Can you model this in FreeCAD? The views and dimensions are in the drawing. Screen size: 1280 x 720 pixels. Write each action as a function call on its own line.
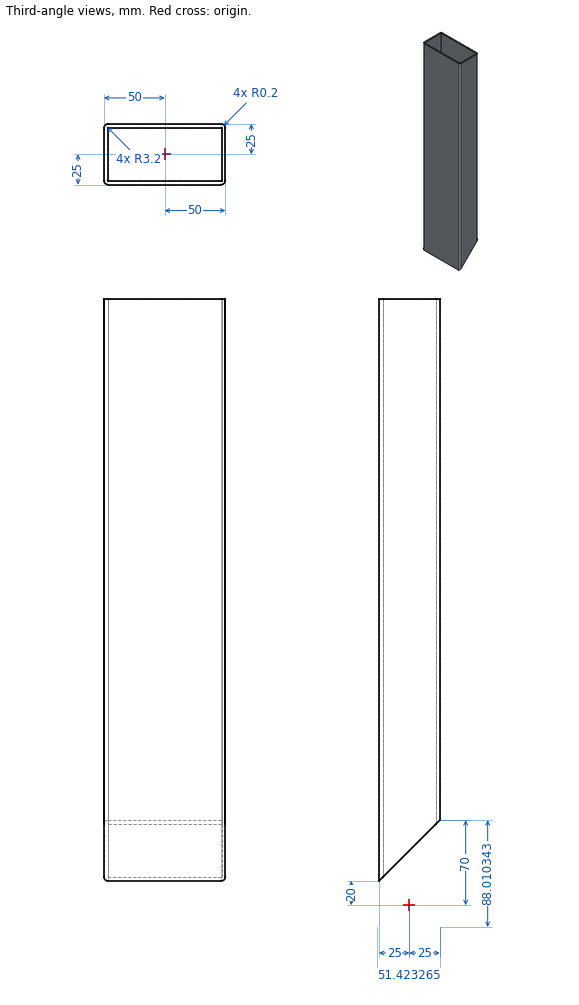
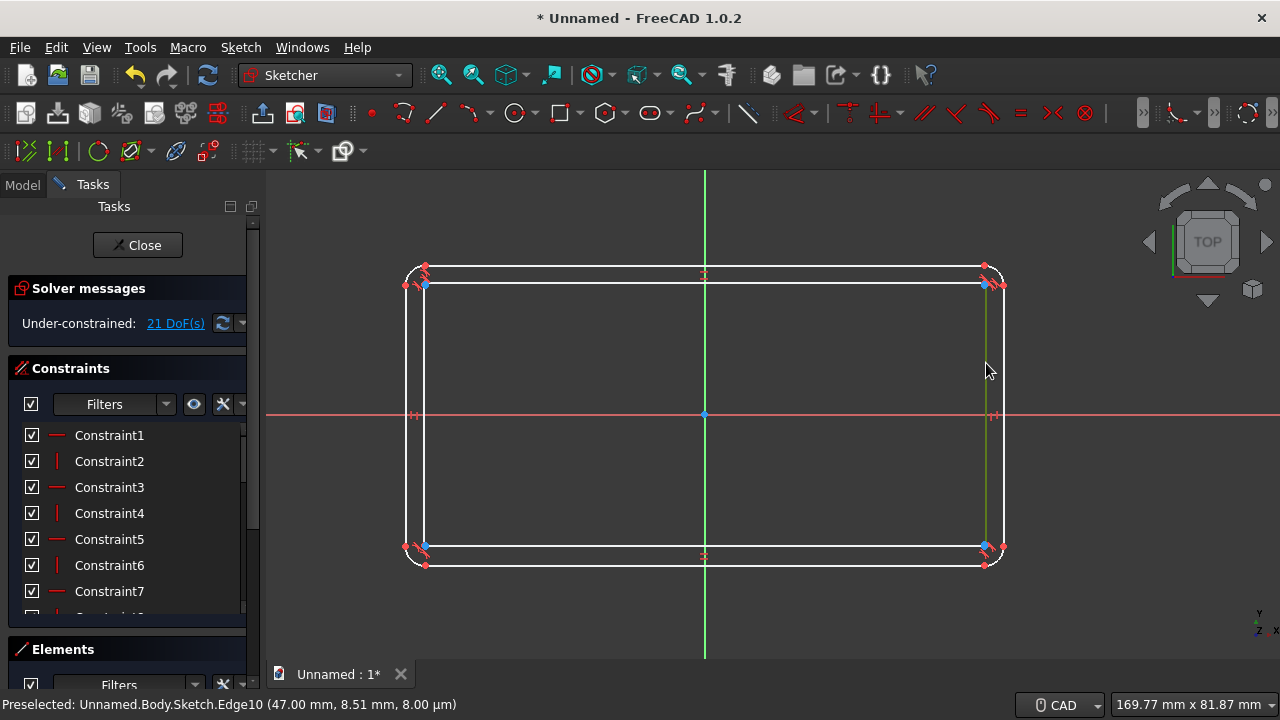
scroll(985, 546, up, 13)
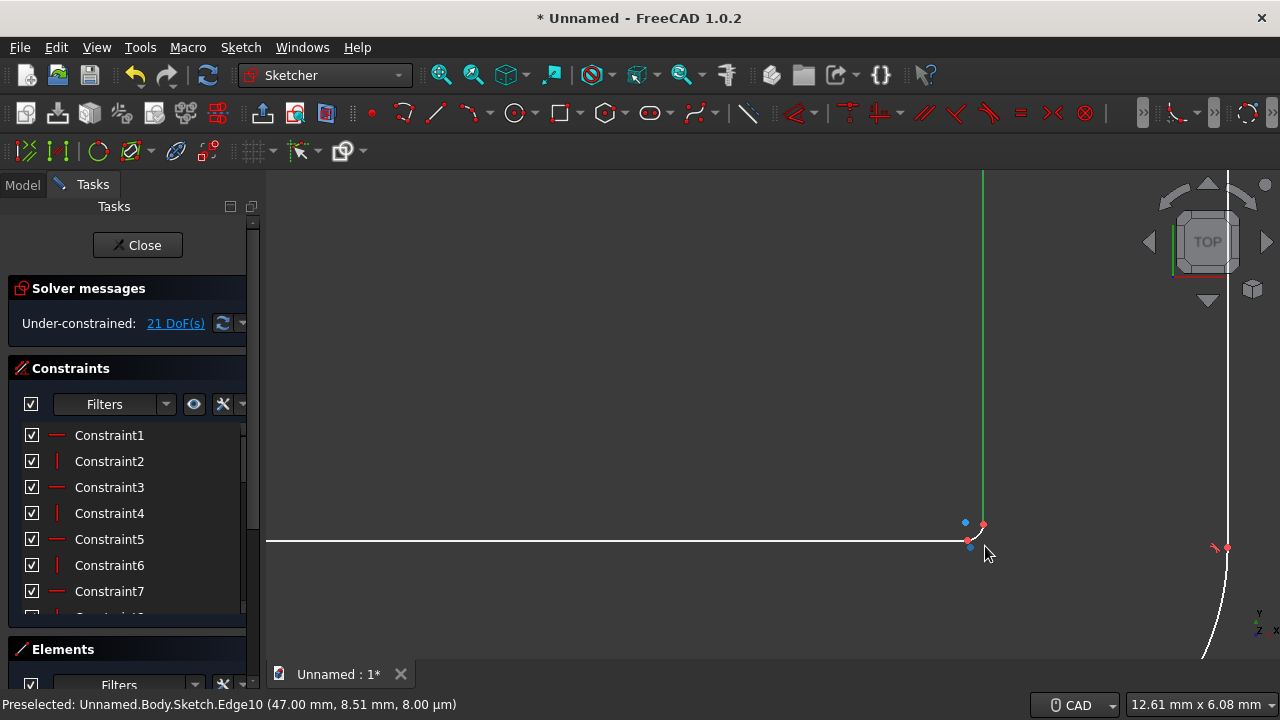
click(978, 536)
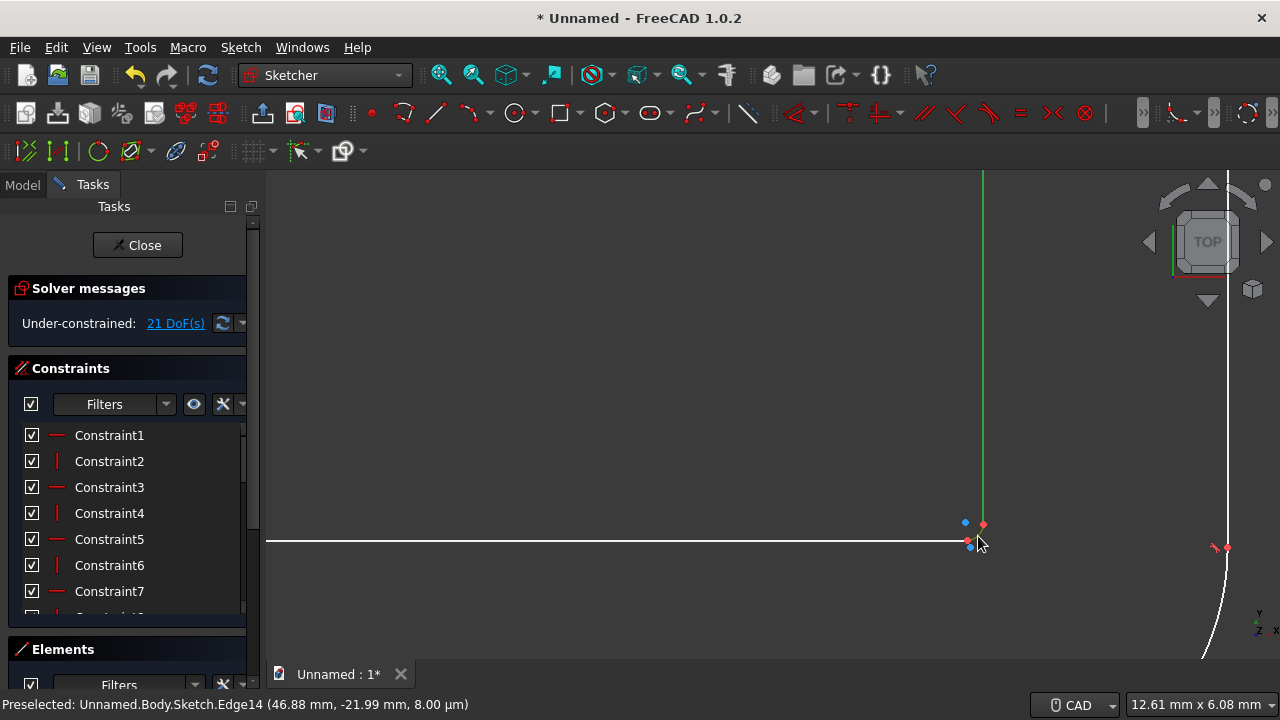
click(990, 114)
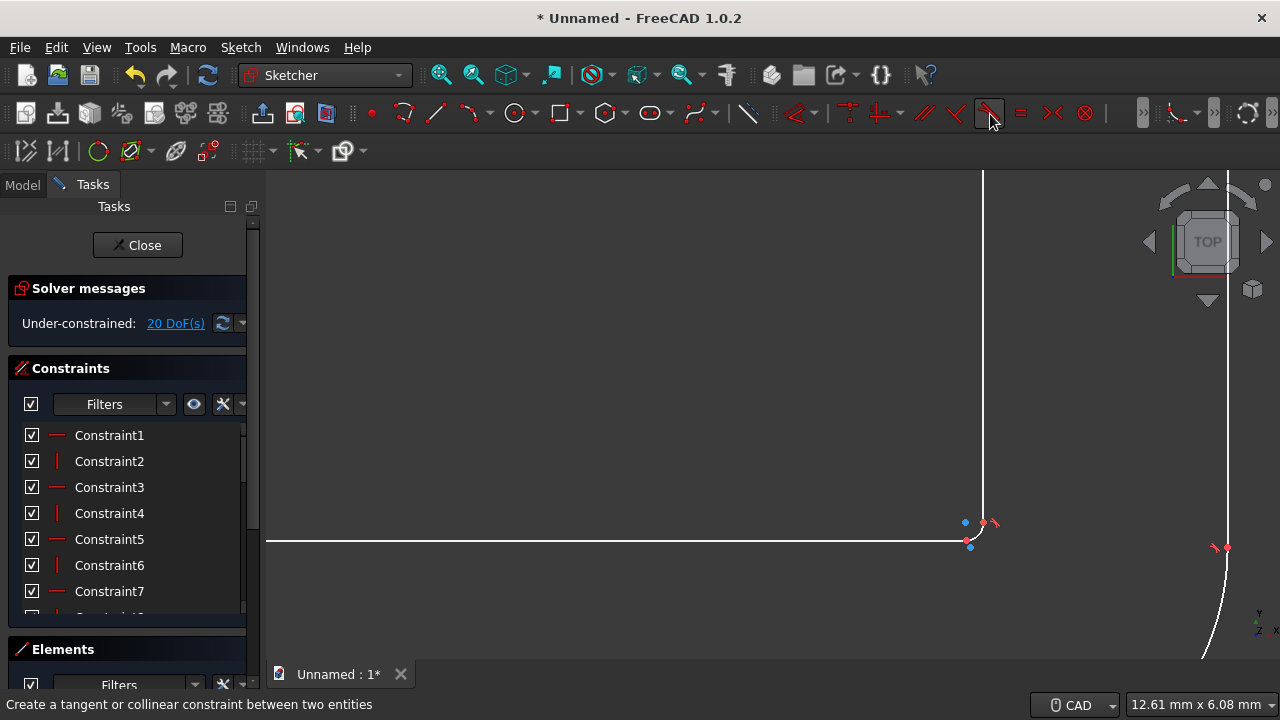
scroll(985, 546, down, 13)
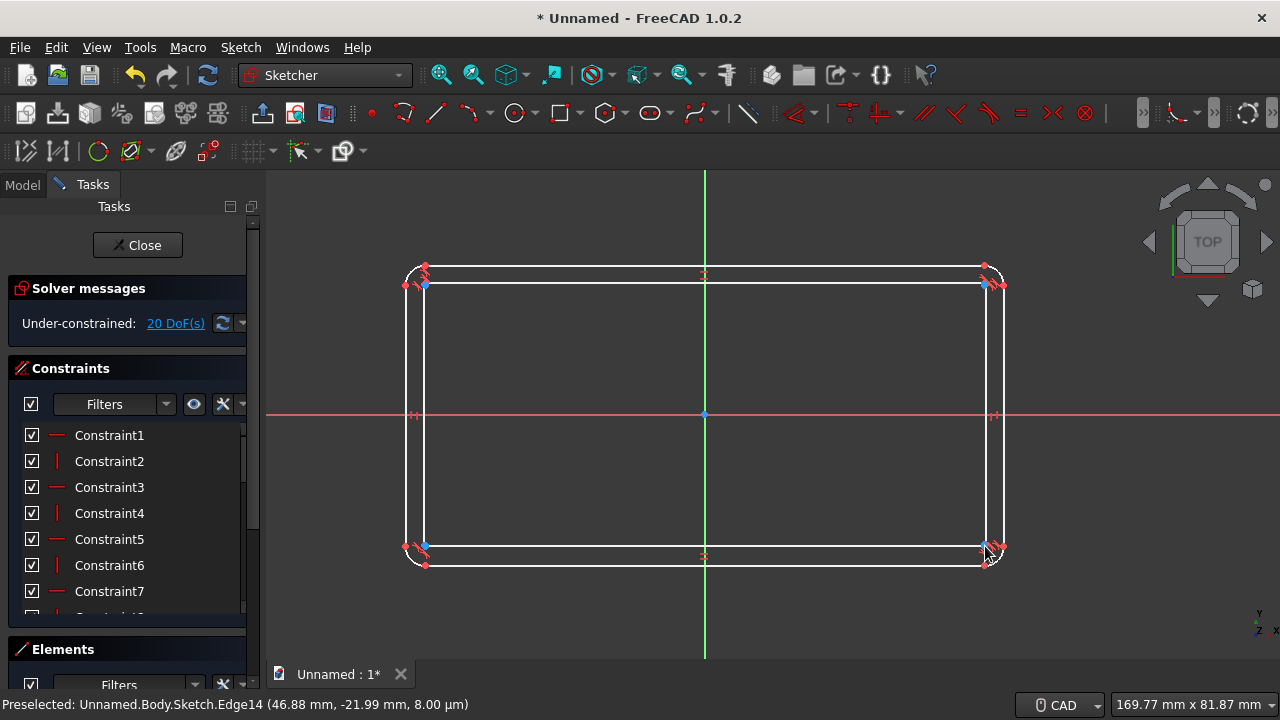
click(817, 546)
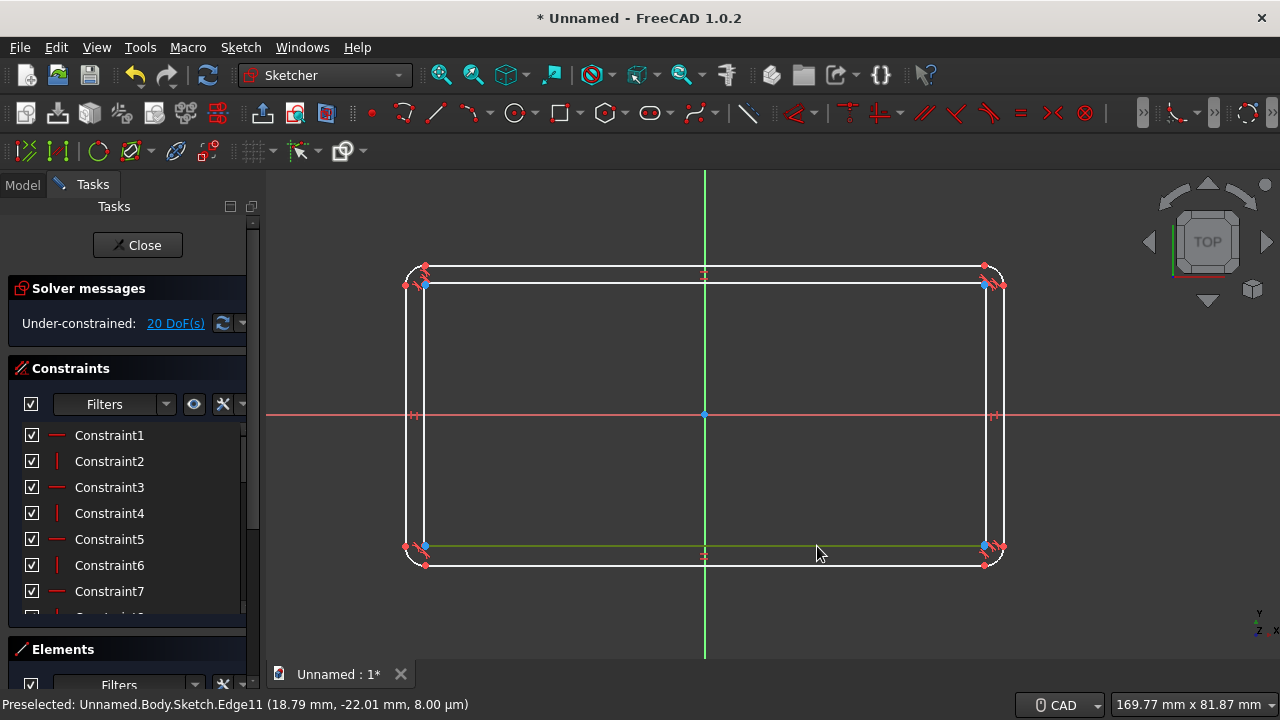
scroll(985, 546, up, 13)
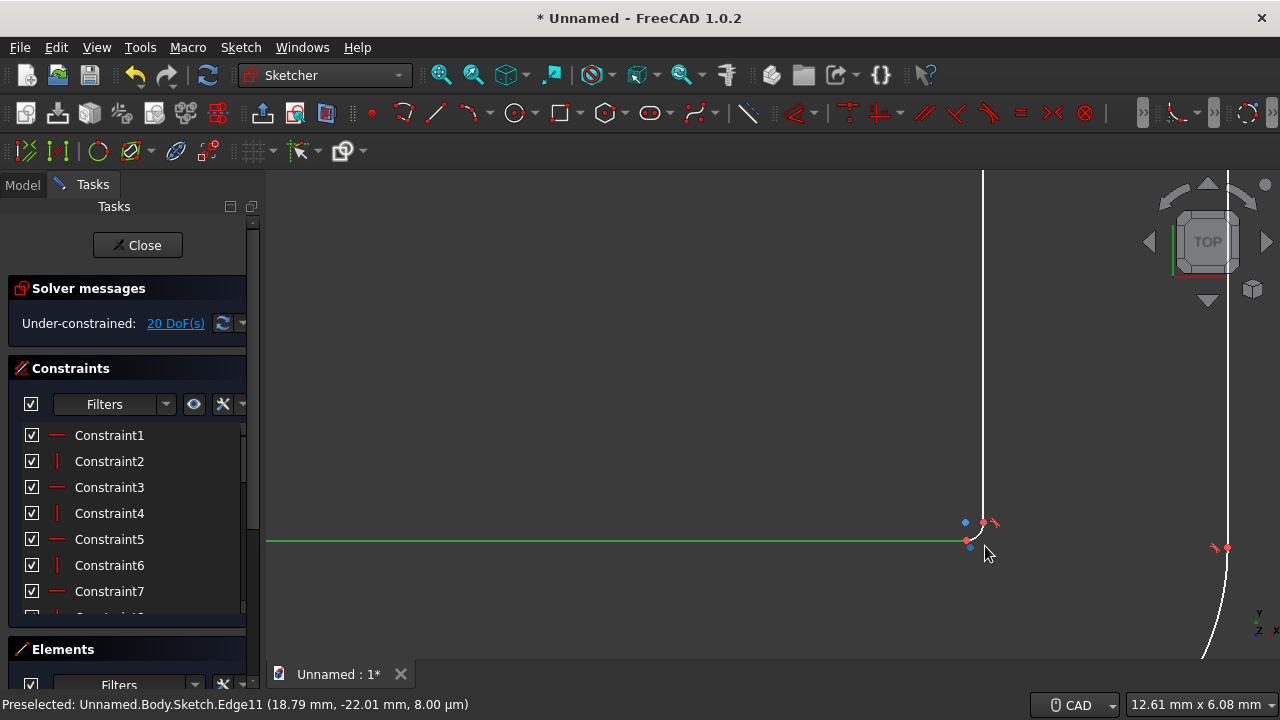
click(979, 535)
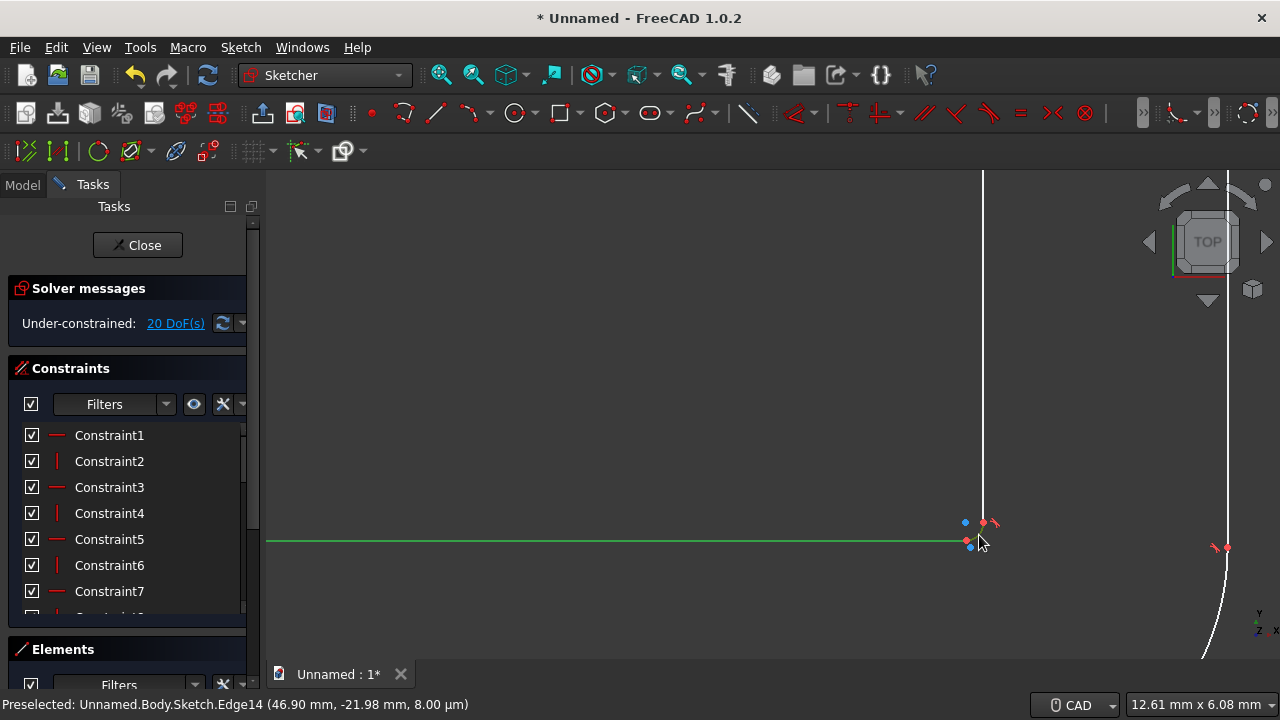
click(990, 114)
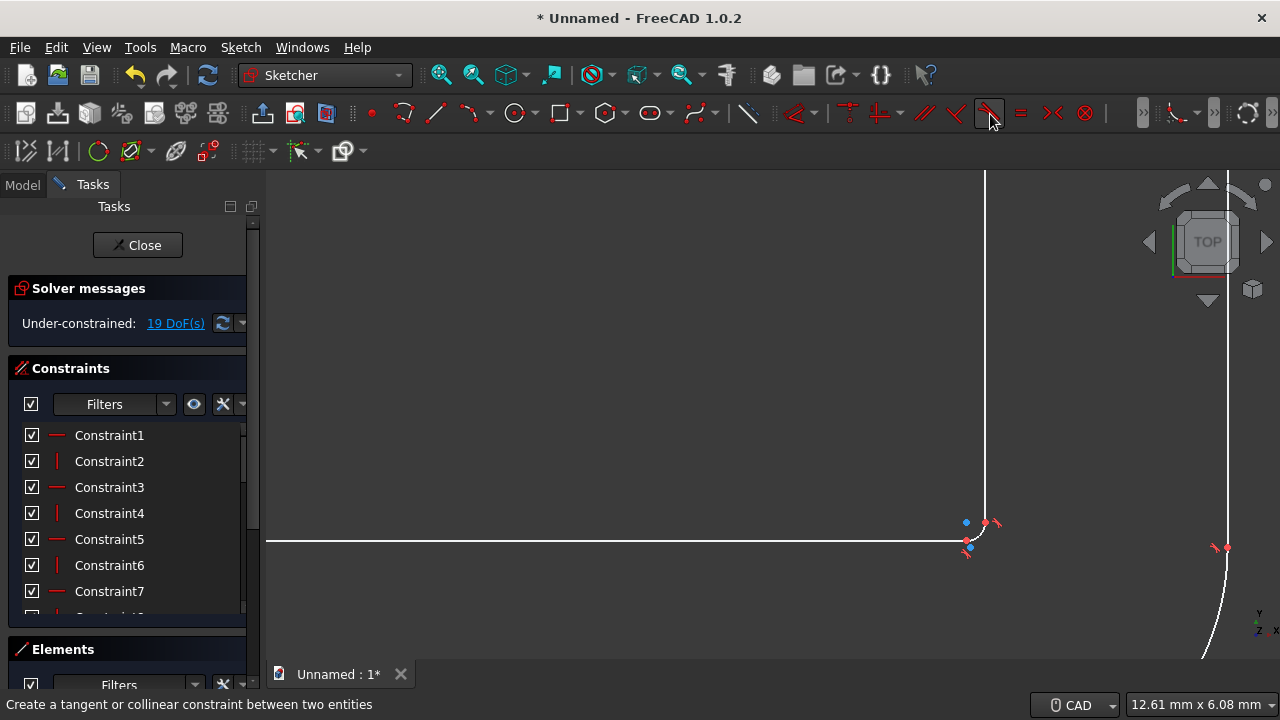
scroll(985, 546, down, 13)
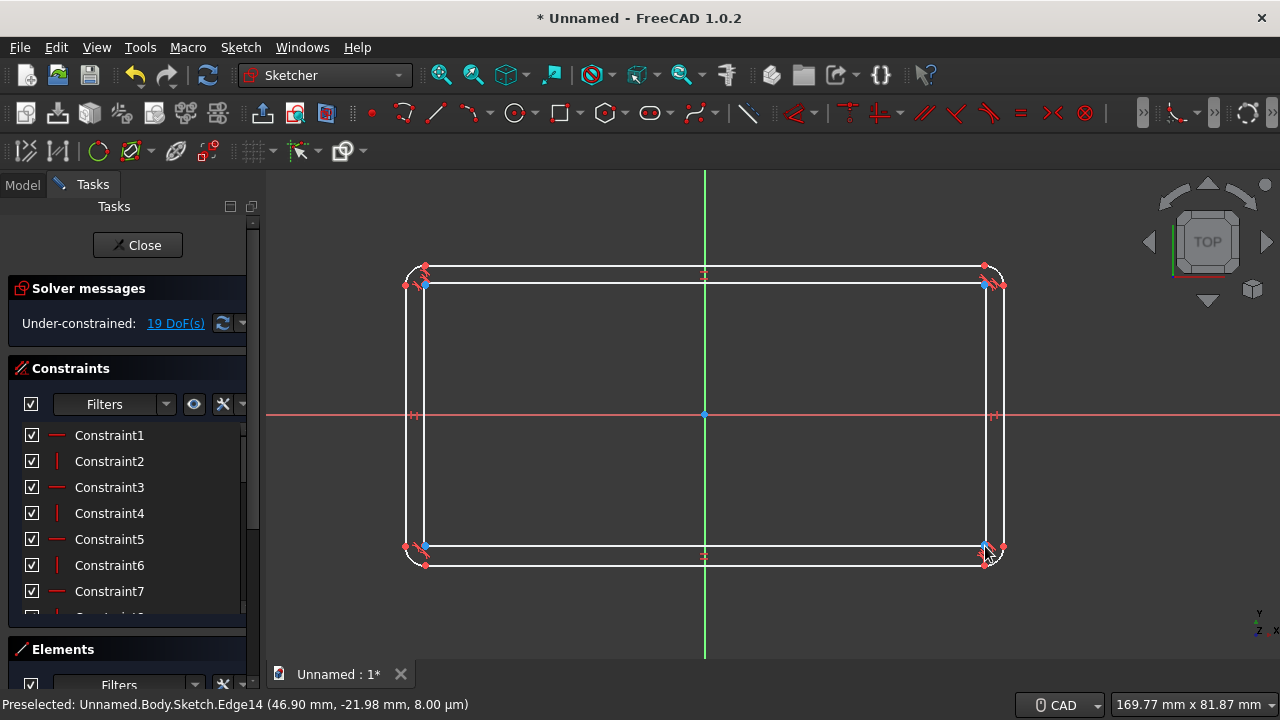
click(817, 546)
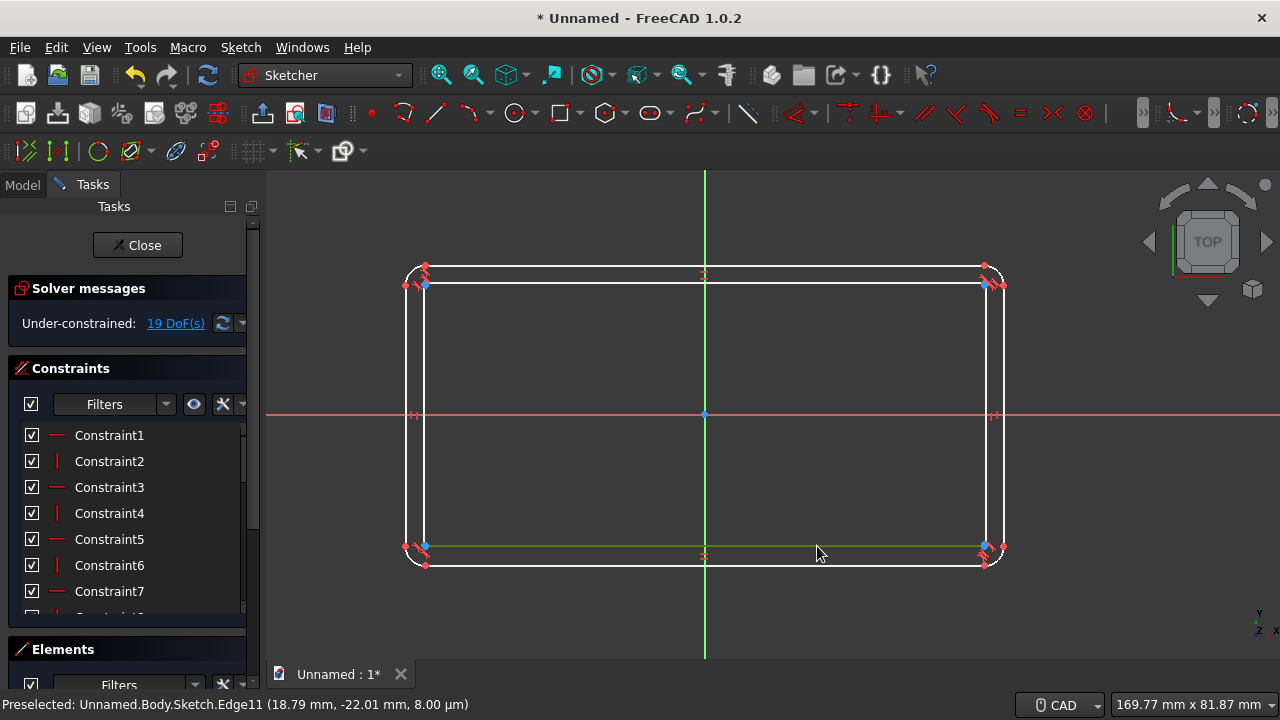
scroll(424, 546, up, 13)